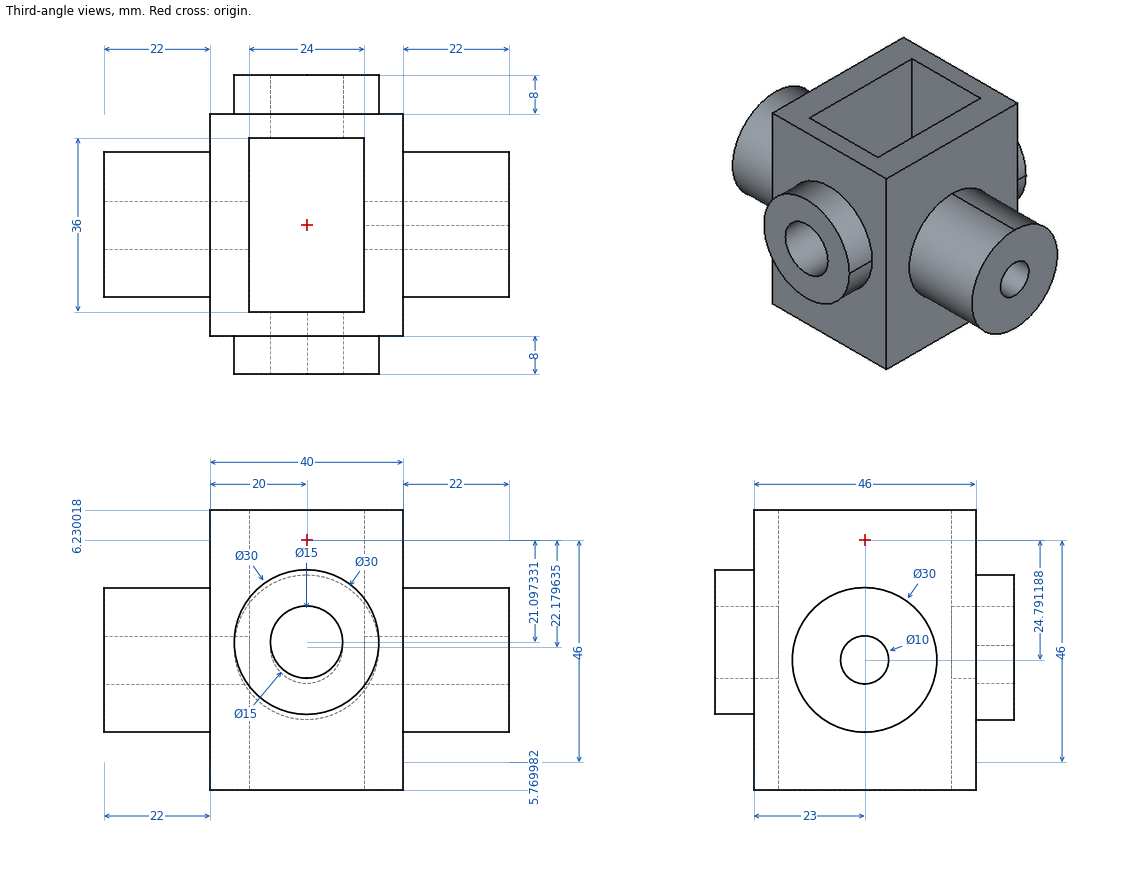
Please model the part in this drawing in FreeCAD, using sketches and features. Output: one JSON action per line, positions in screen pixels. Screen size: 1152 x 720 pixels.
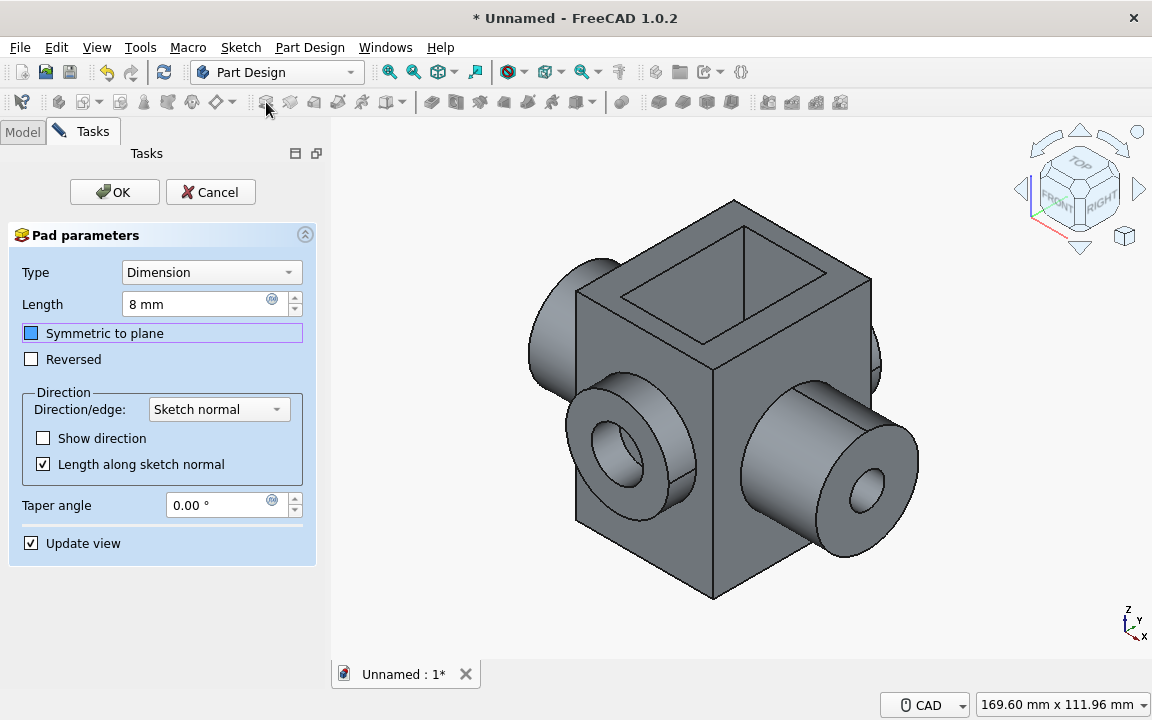
{"action": "left_click", "coordinate": [115, 192]}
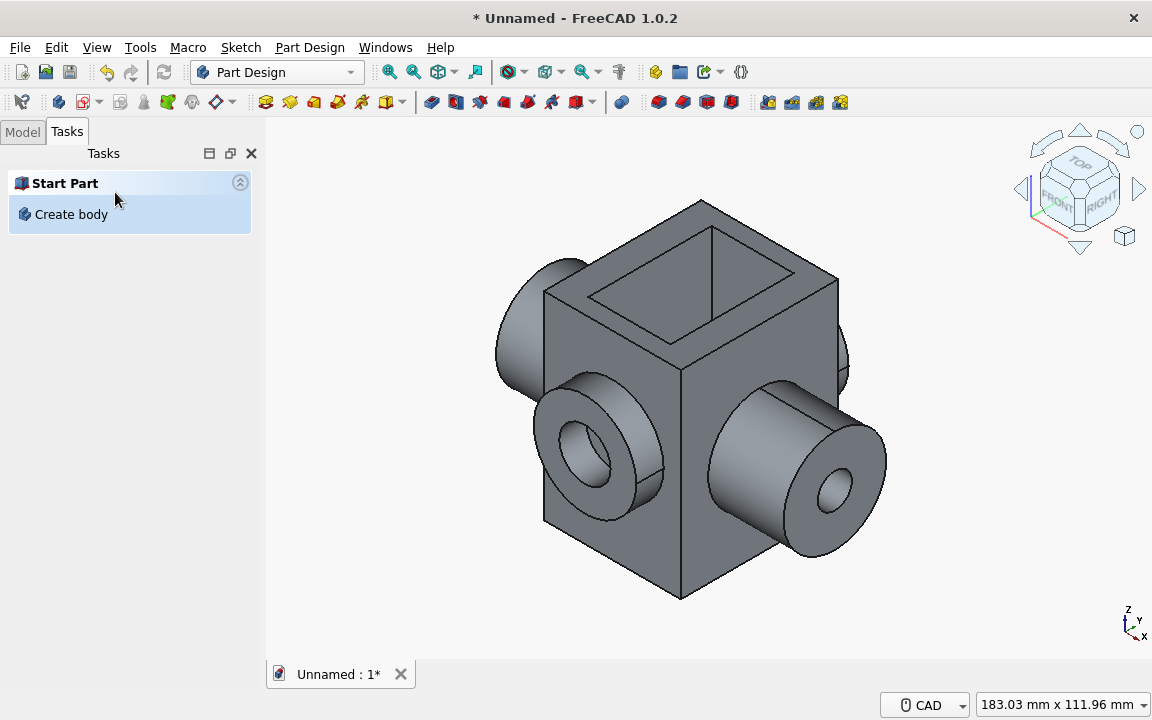
{"action": "left_click", "coordinate": [23, 131]}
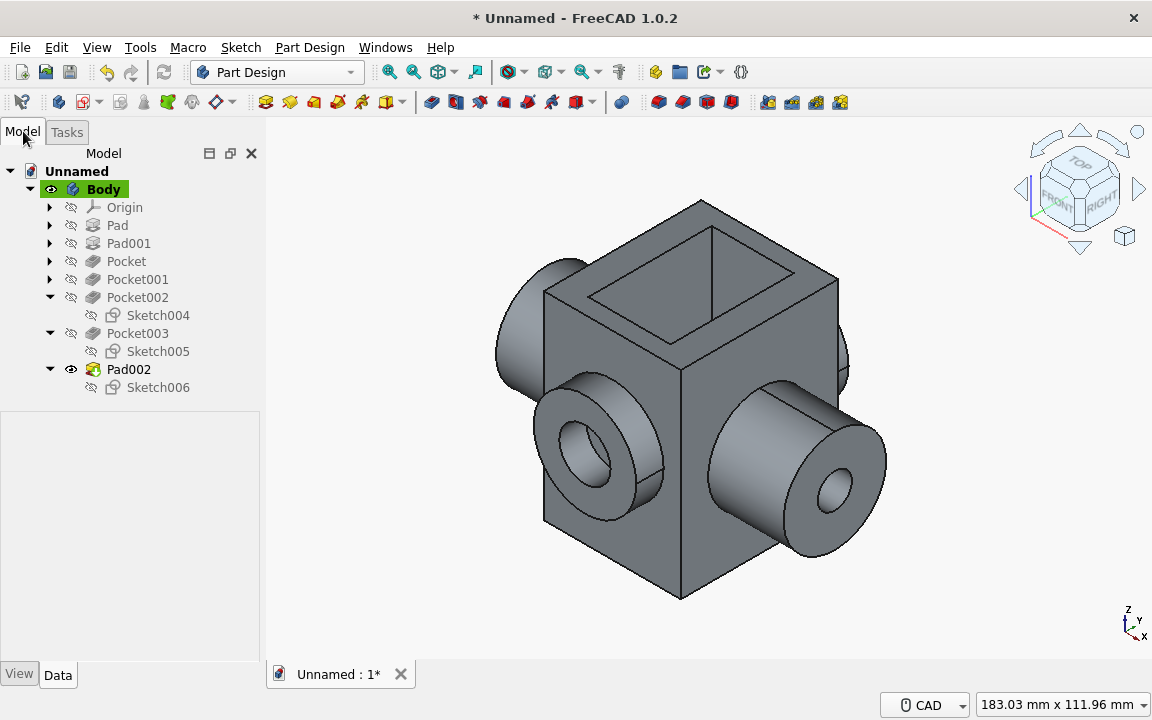
{"action": "left_click", "coordinate": [50, 207]}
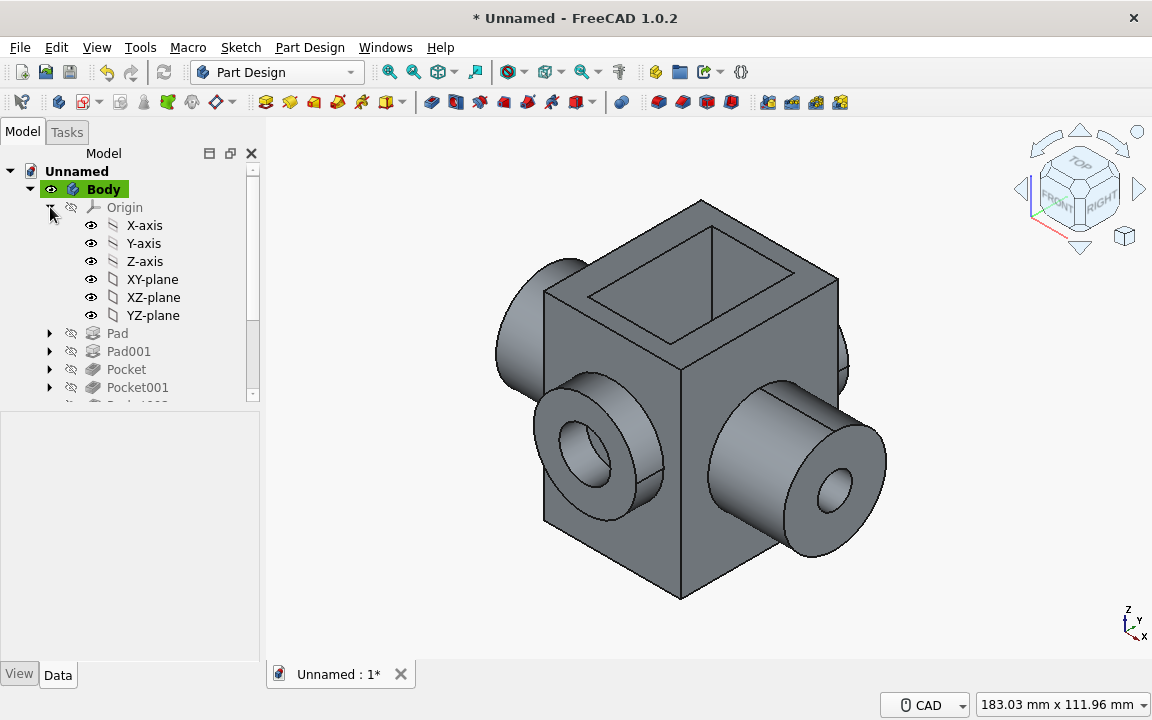
{"action": "left_click", "coordinate": [136, 297]}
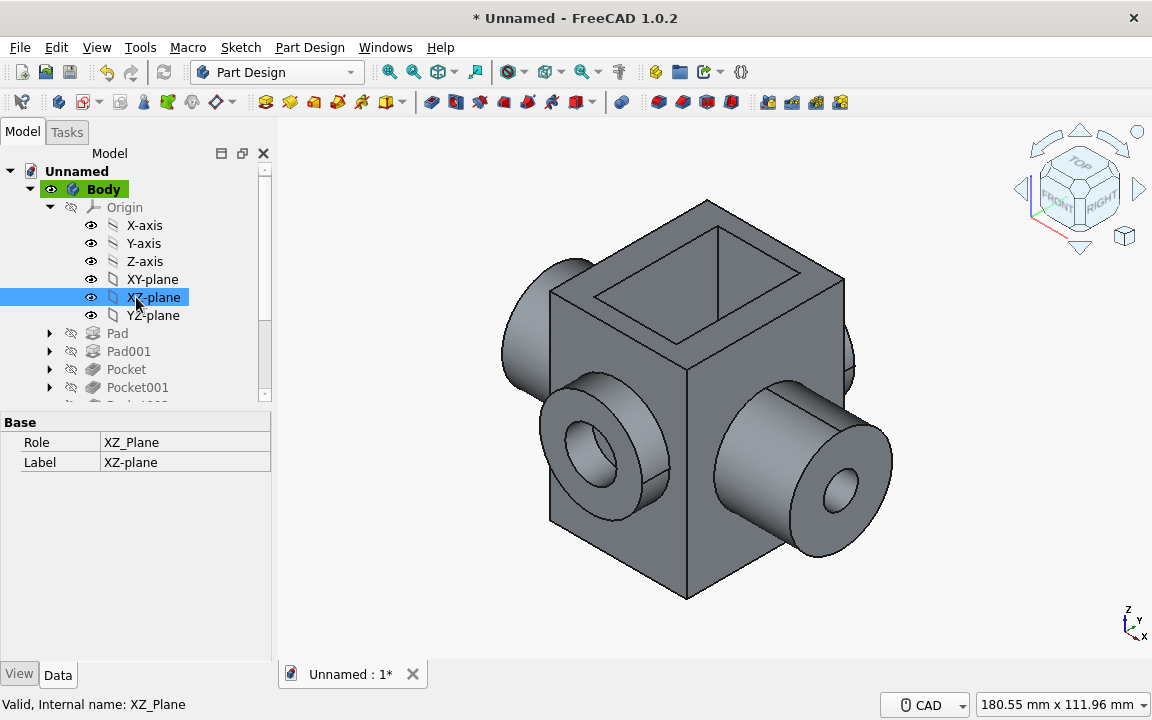
{"action": "left_click", "coordinate": [216, 102]}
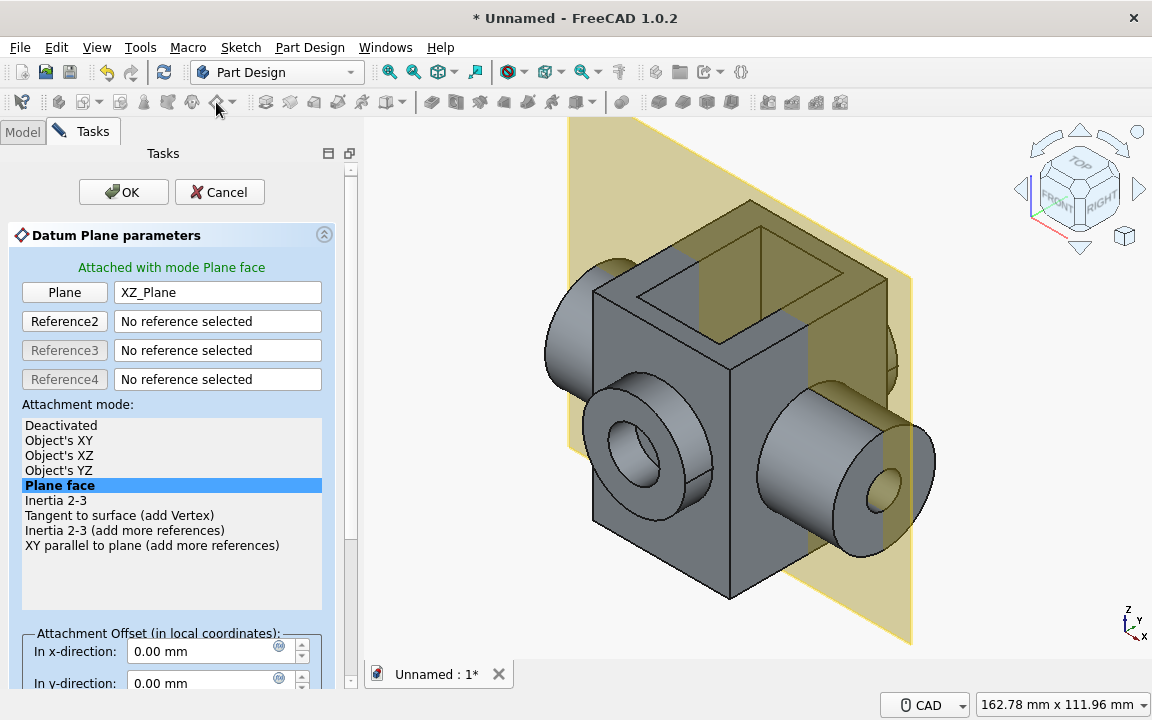
{"action": "scroll", "coordinate": [351, 426], "scroll_direction": "down", "scroll_amount": 2}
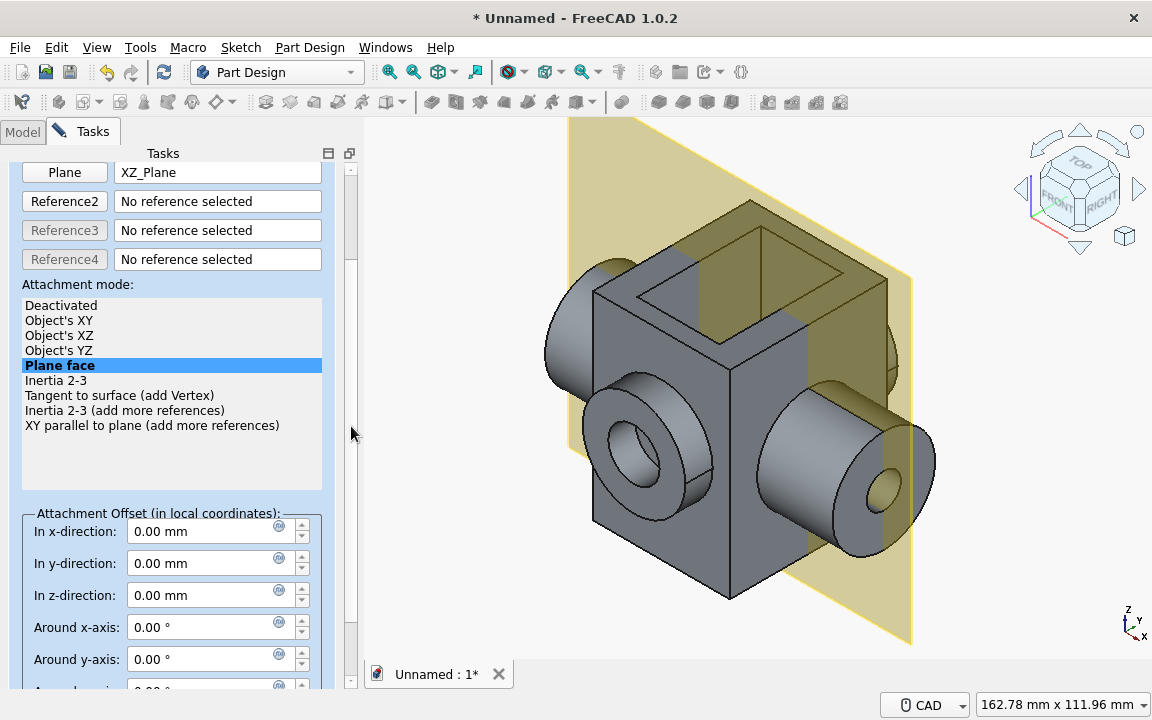
{"action": "triple_click", "coordinate": [210, 595]}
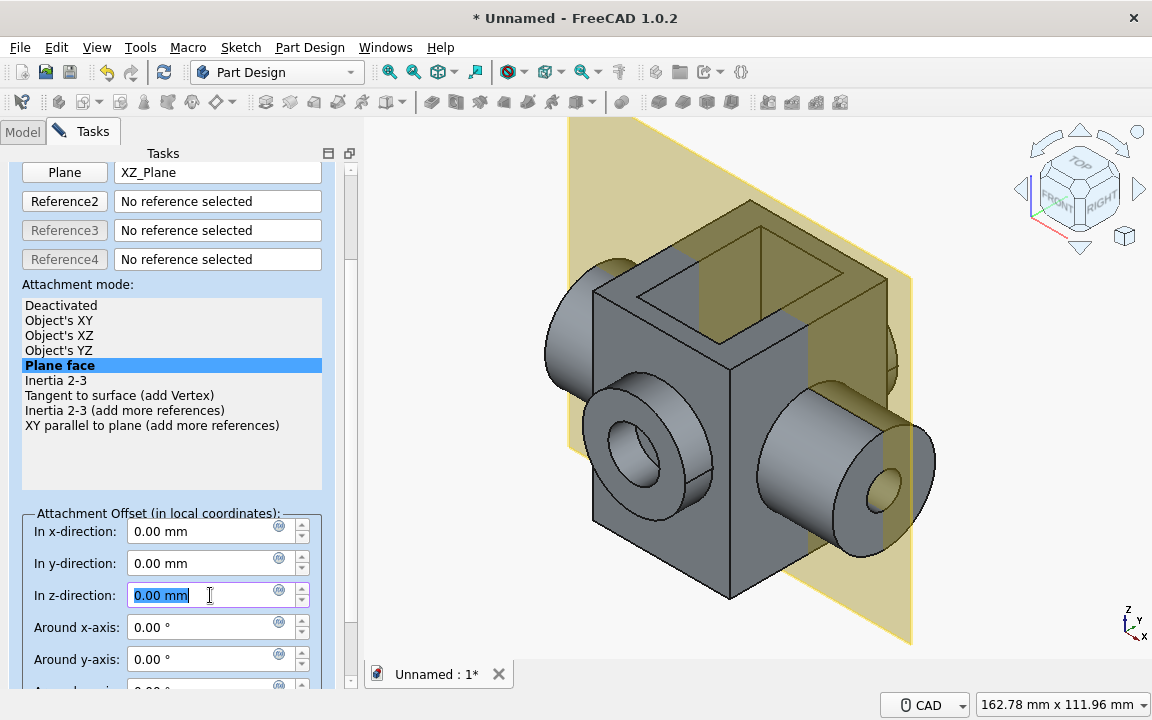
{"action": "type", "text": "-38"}
{"action": "key", "text": "Tab"}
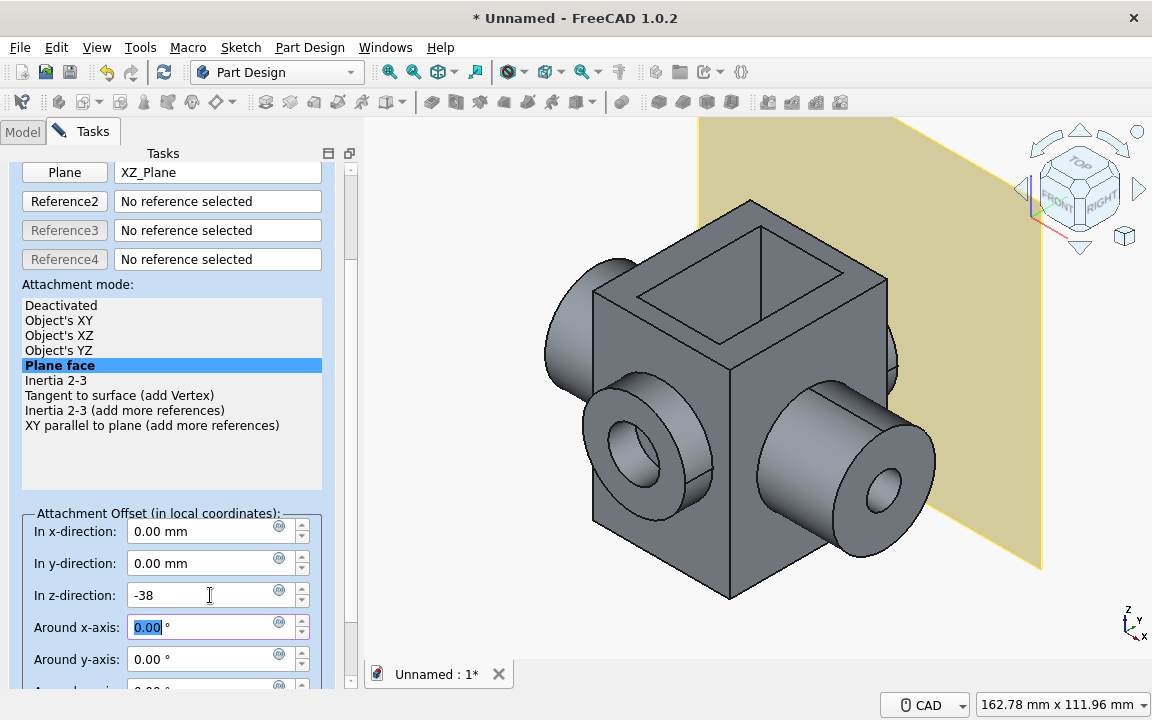
{"action": "scroll", "coordinate": [351, 426], "scroll_direction": "up", "scroll_amount": 3}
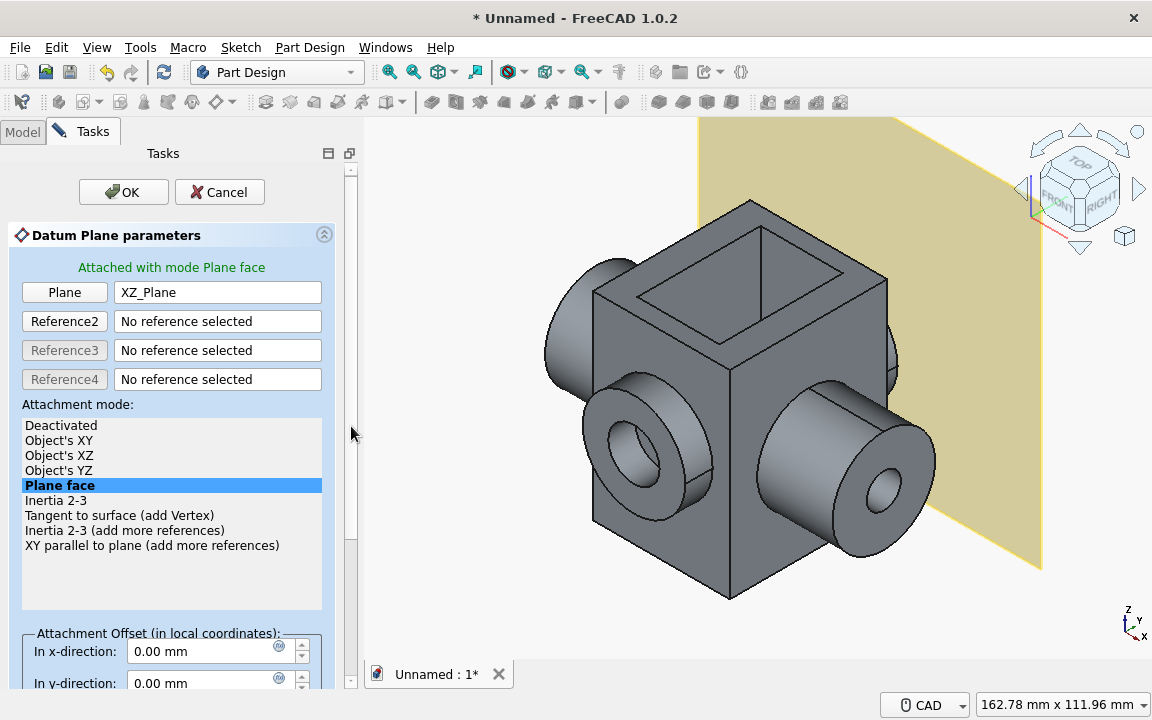
{"action": "left_click", "coordinate": [124, 192]}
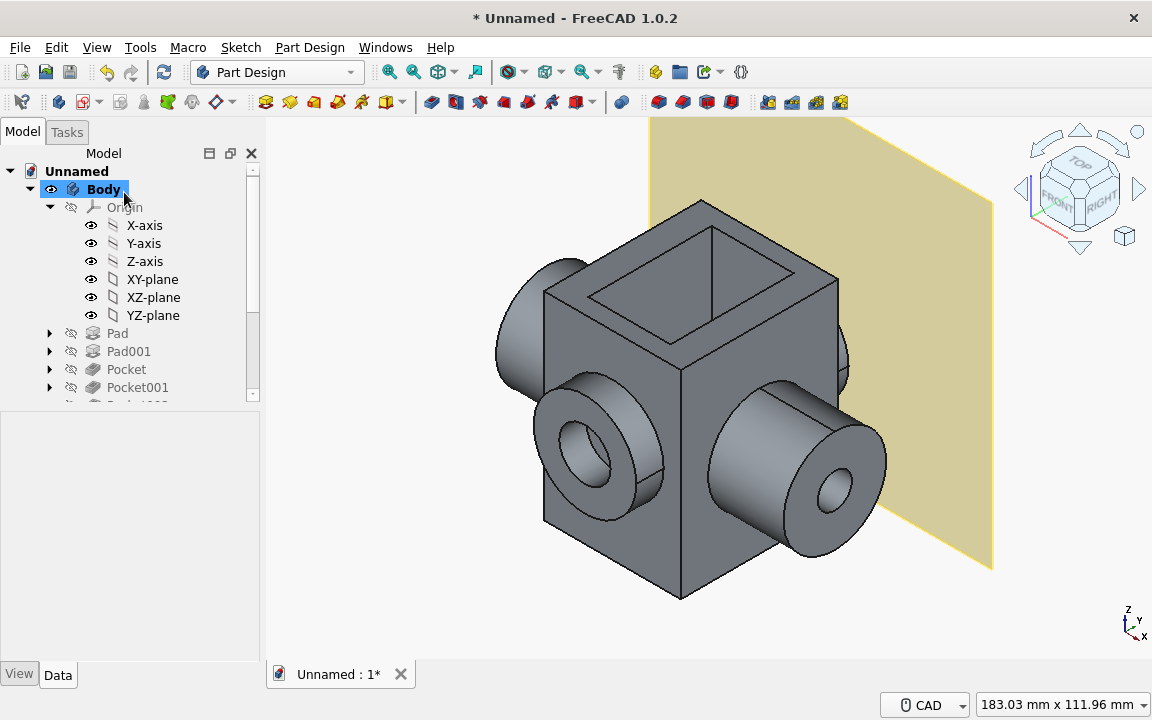
{"action": "scroll", "coordinate": [100, 275], "scroll_direction": "down", "scroll_amount": 3}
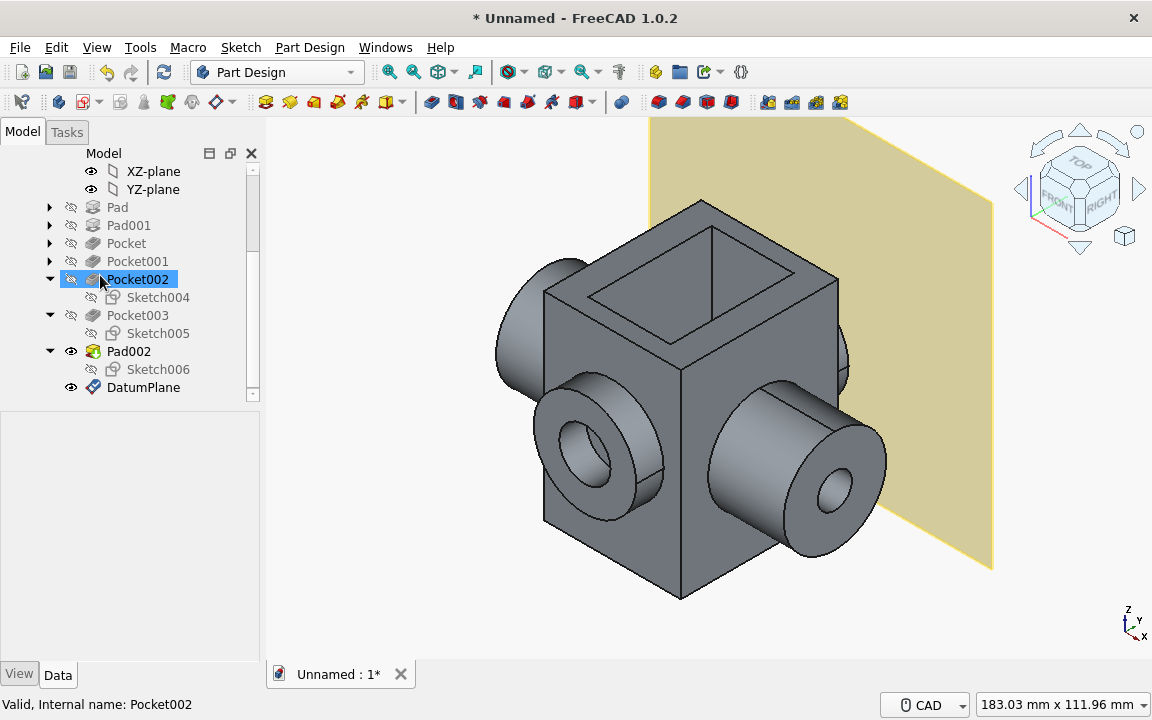
{"action": "left_click", "coordinate": [116, 387]}